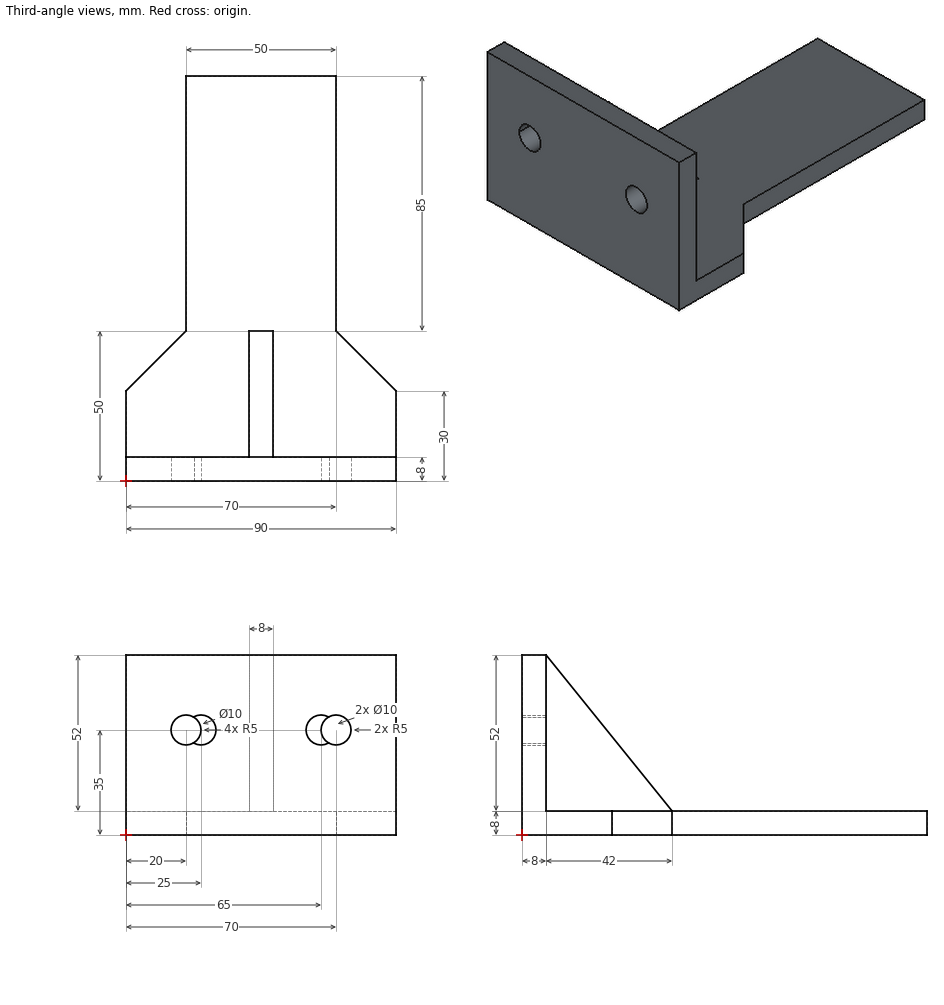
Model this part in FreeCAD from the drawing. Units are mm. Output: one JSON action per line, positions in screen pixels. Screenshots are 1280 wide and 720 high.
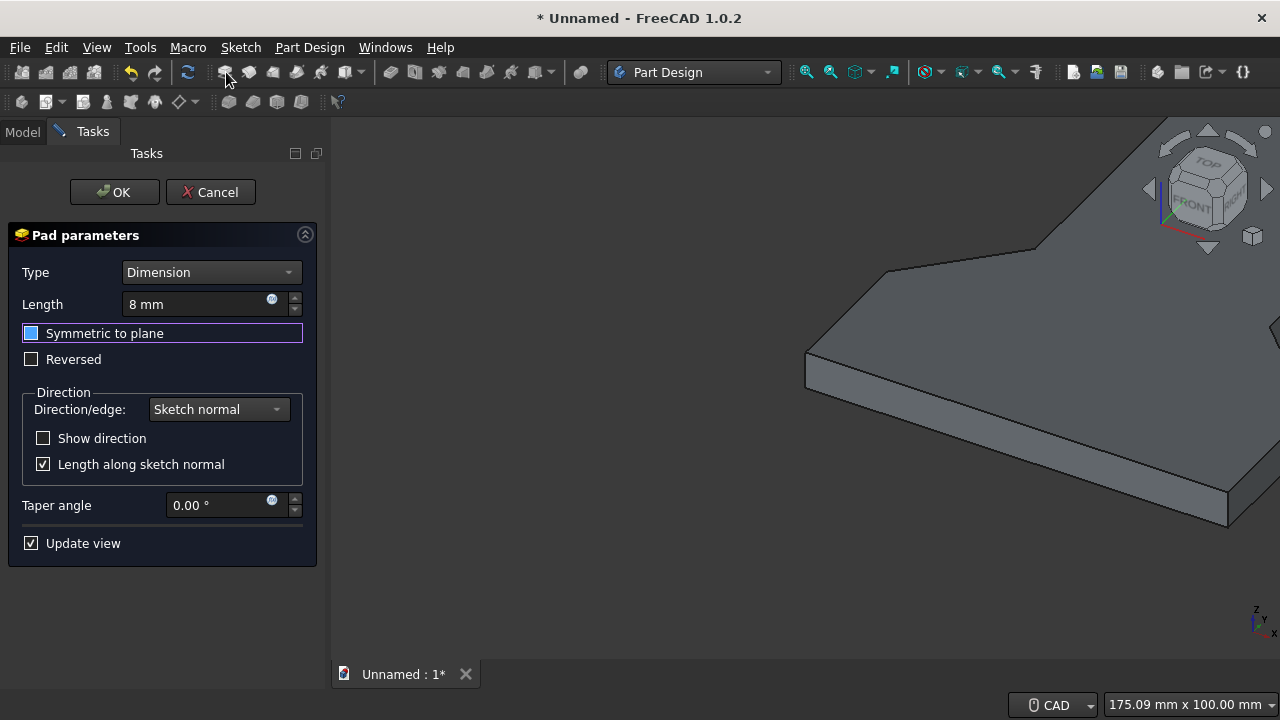
{"action": "left_click", "coordinate": [115, 192]}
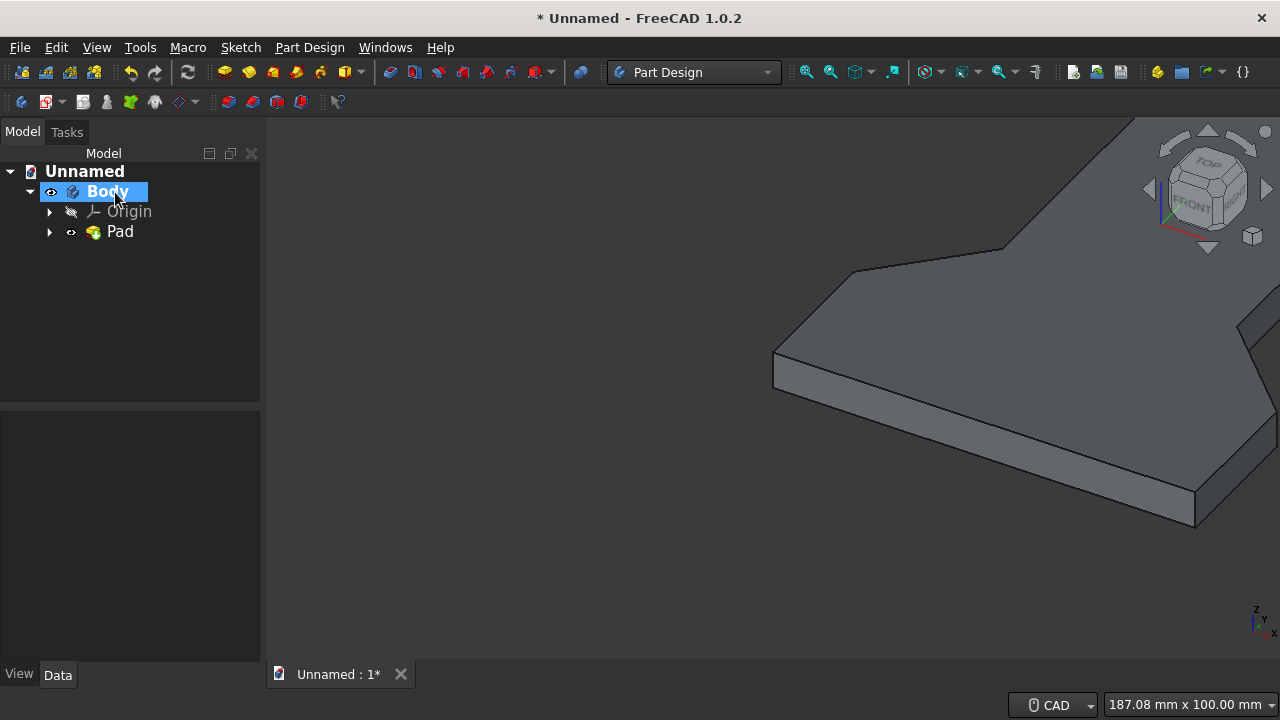
{"action": "left_click", "coordinate": [808, 72]}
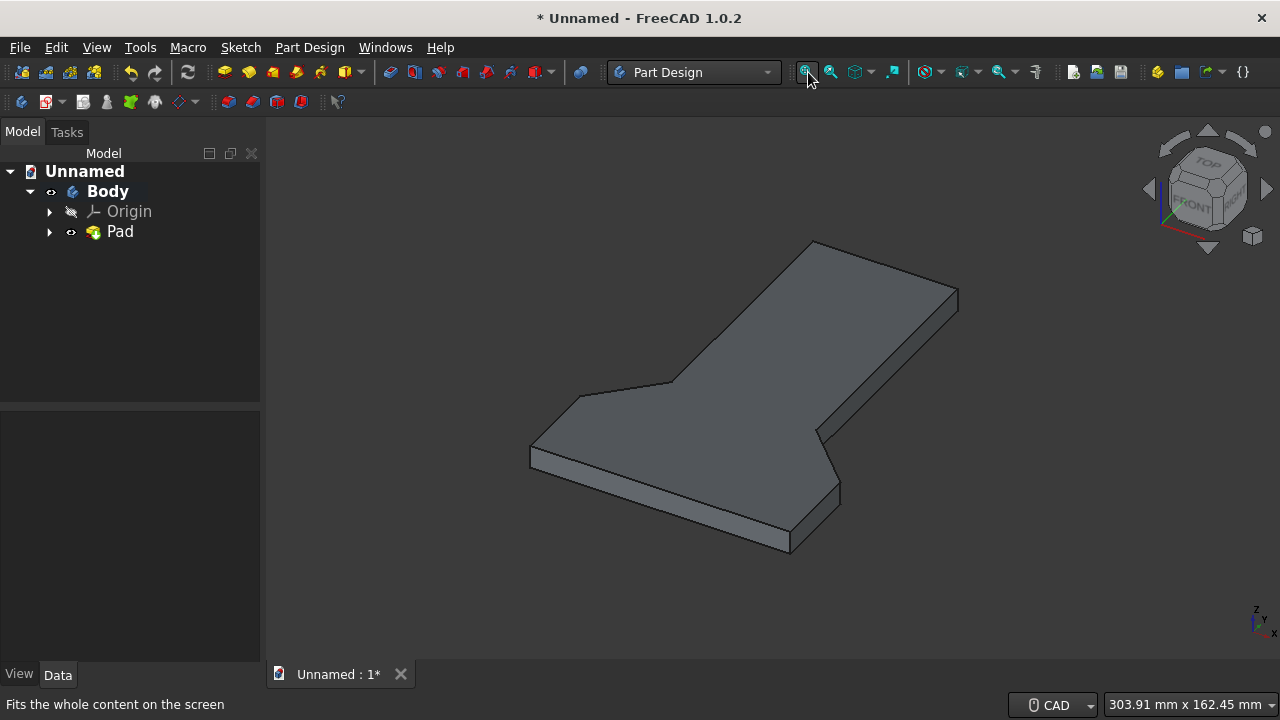
{"action": "left_click", "coordinate": [709, 440]}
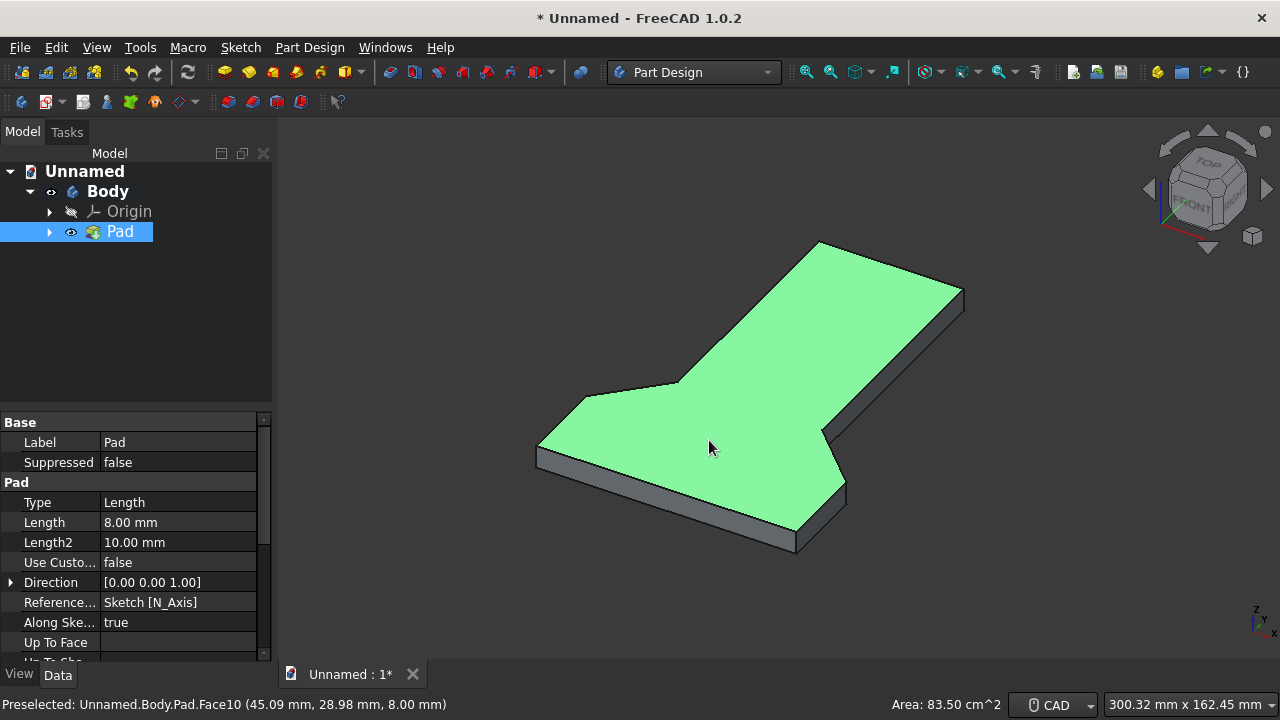
{"action": "left_click", "coordinate": [46, 102]}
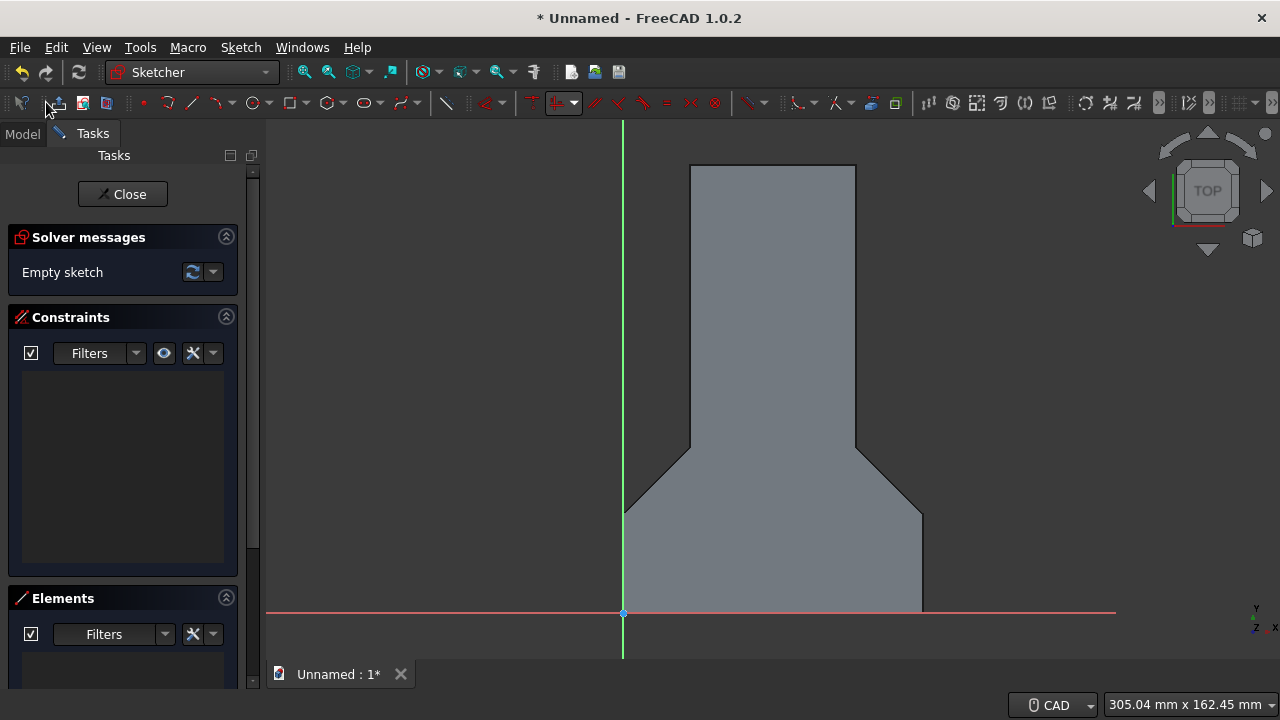
{"action": "scroll", "coordinate": [856, 631], "scroll_direction": "up", "scroll_amount": 3}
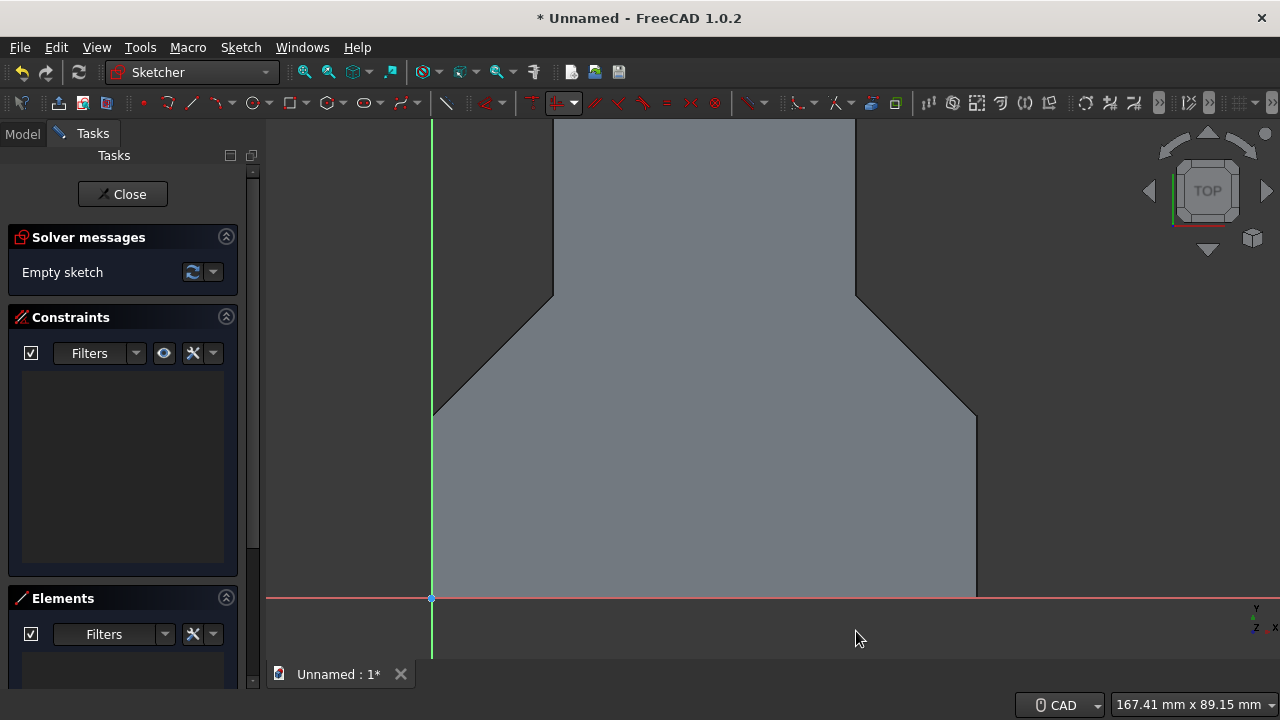
{"action": "left_click", "coordinate": [290, 104]}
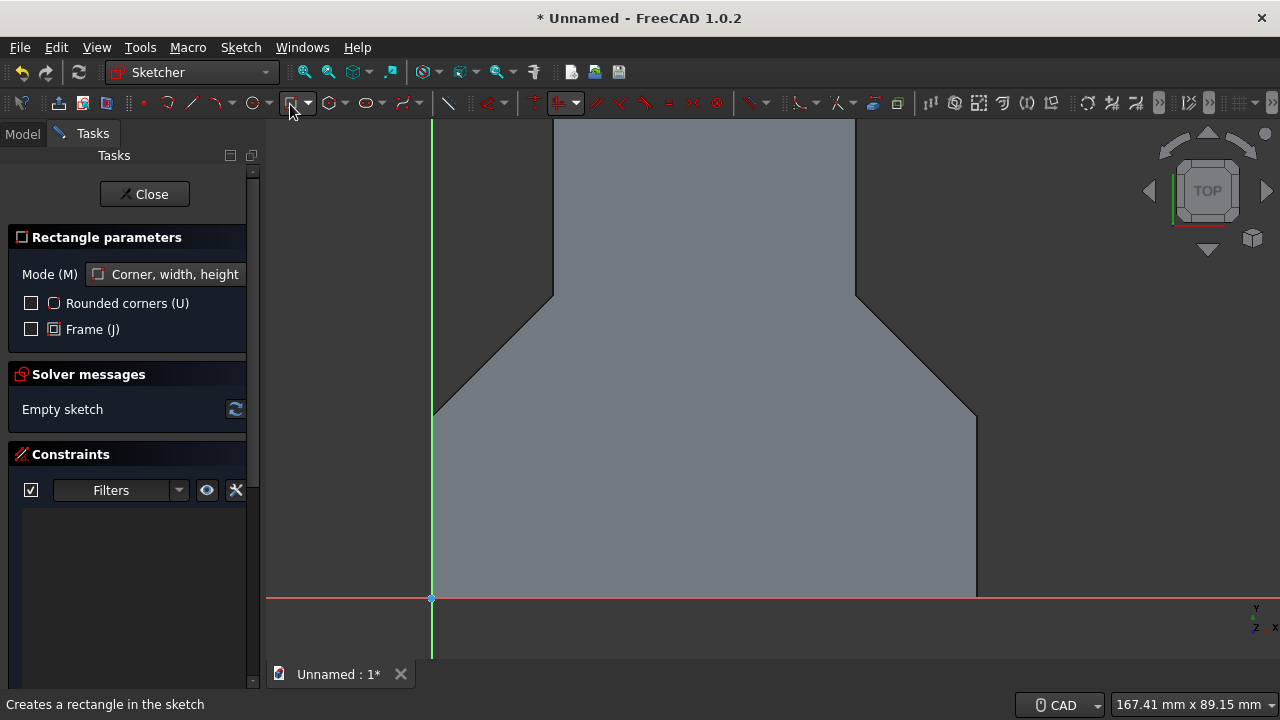
{"action": "left_click", "coordinate": [432, 598]}
{"action": "mouse_move", "coordinate": [977, 550]}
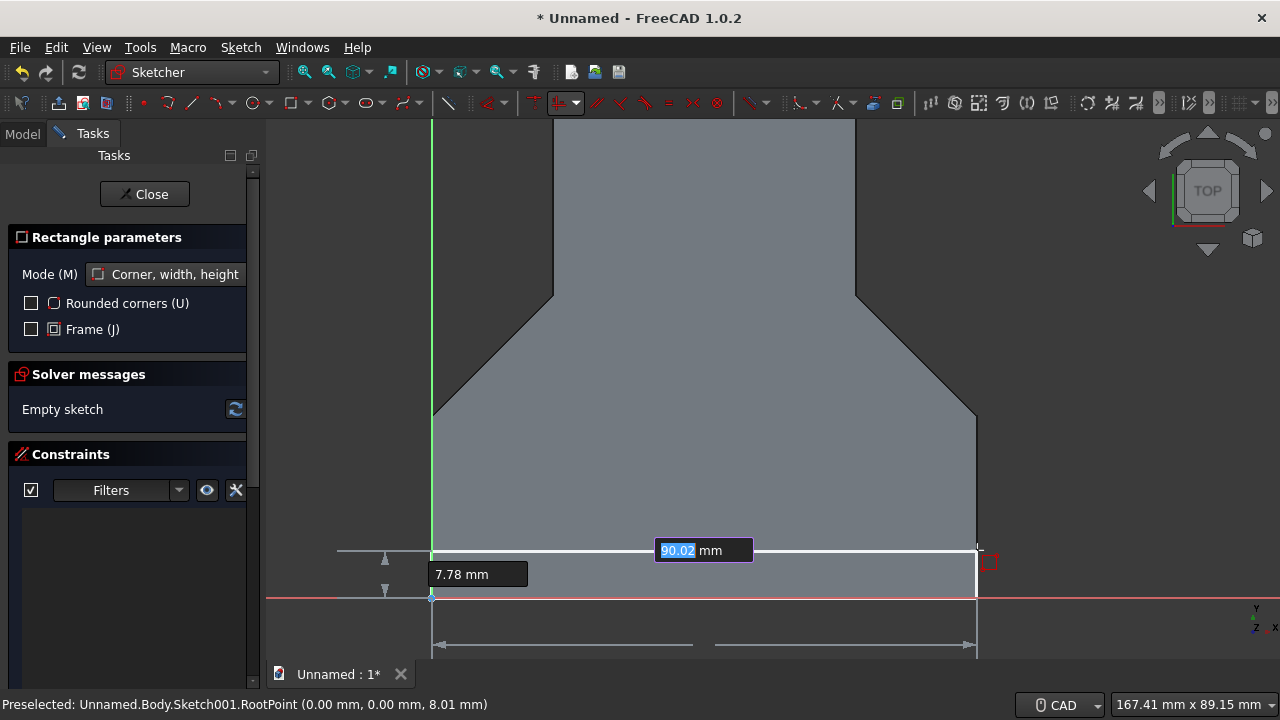
{"action": "type", "text": "90"}
{"action": "key", "text": "Tab"}
{"action": "type", "text": "8"}
{"action": "key", "text": "Return"}
{"action": "key", "text": "Escape"}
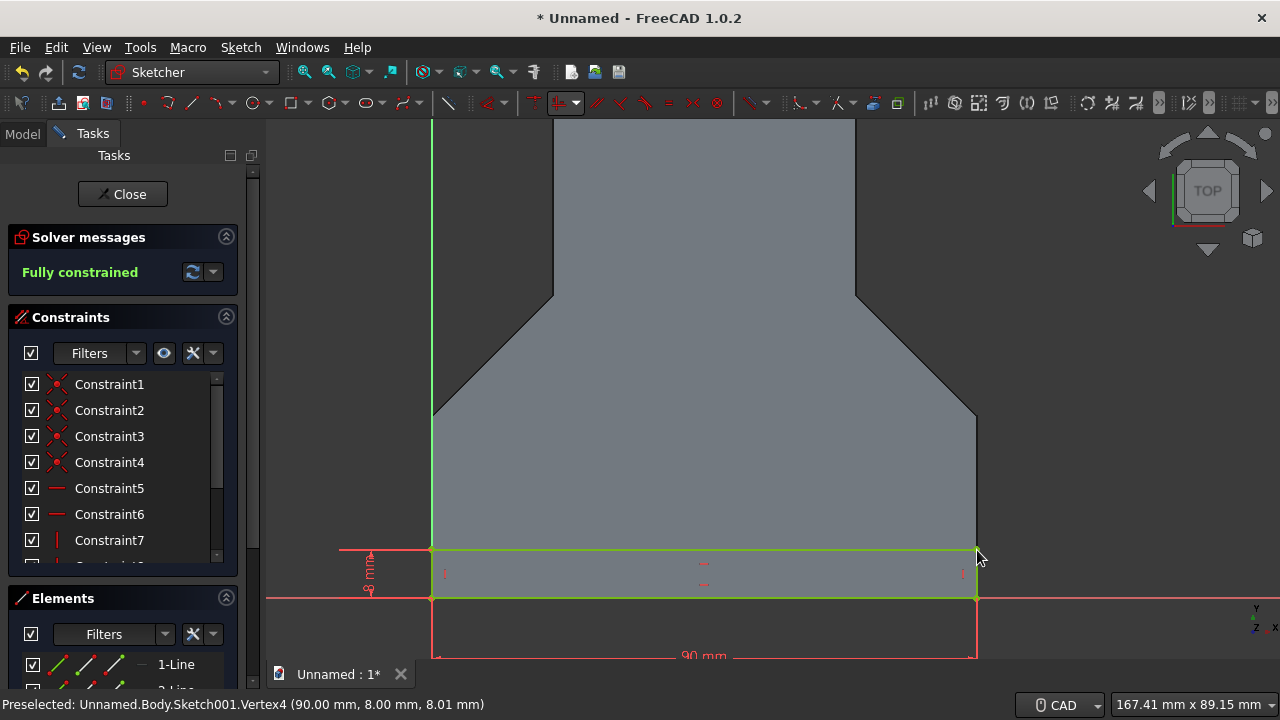
{"action": "left_click", "coordinate": [123, 194]}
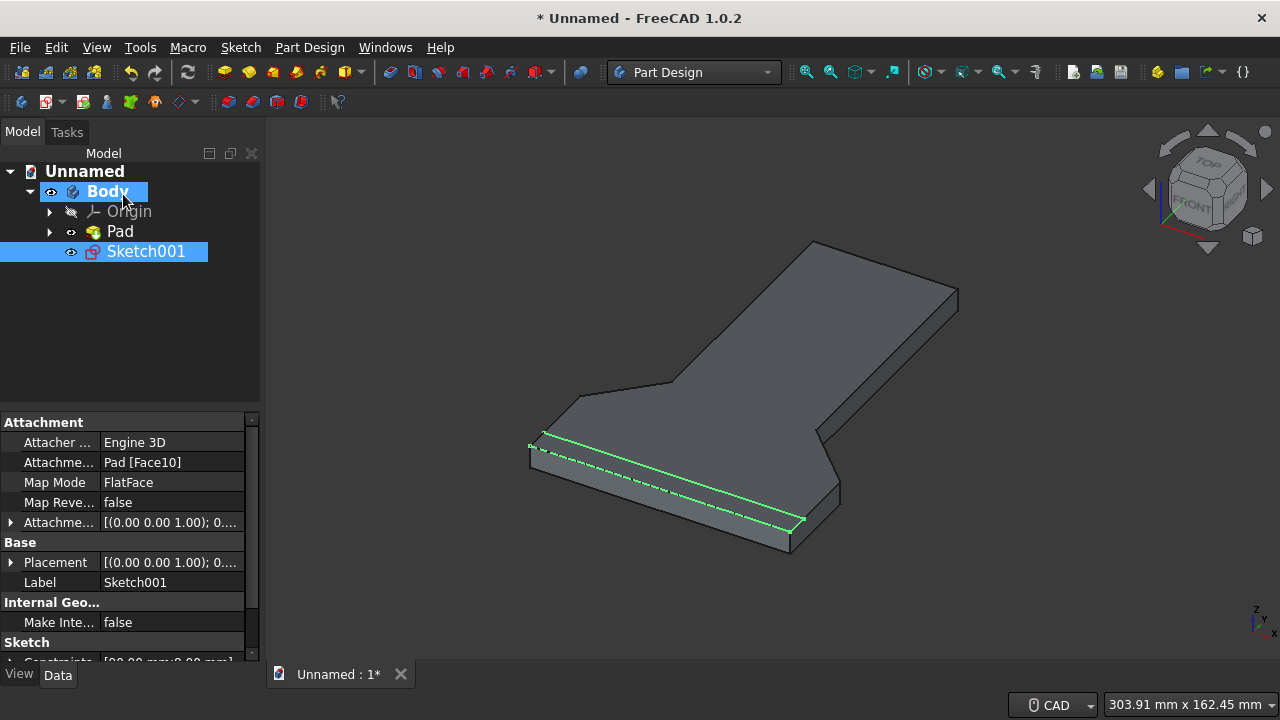
{"action": "left_click", "coordinate": [226, 72]}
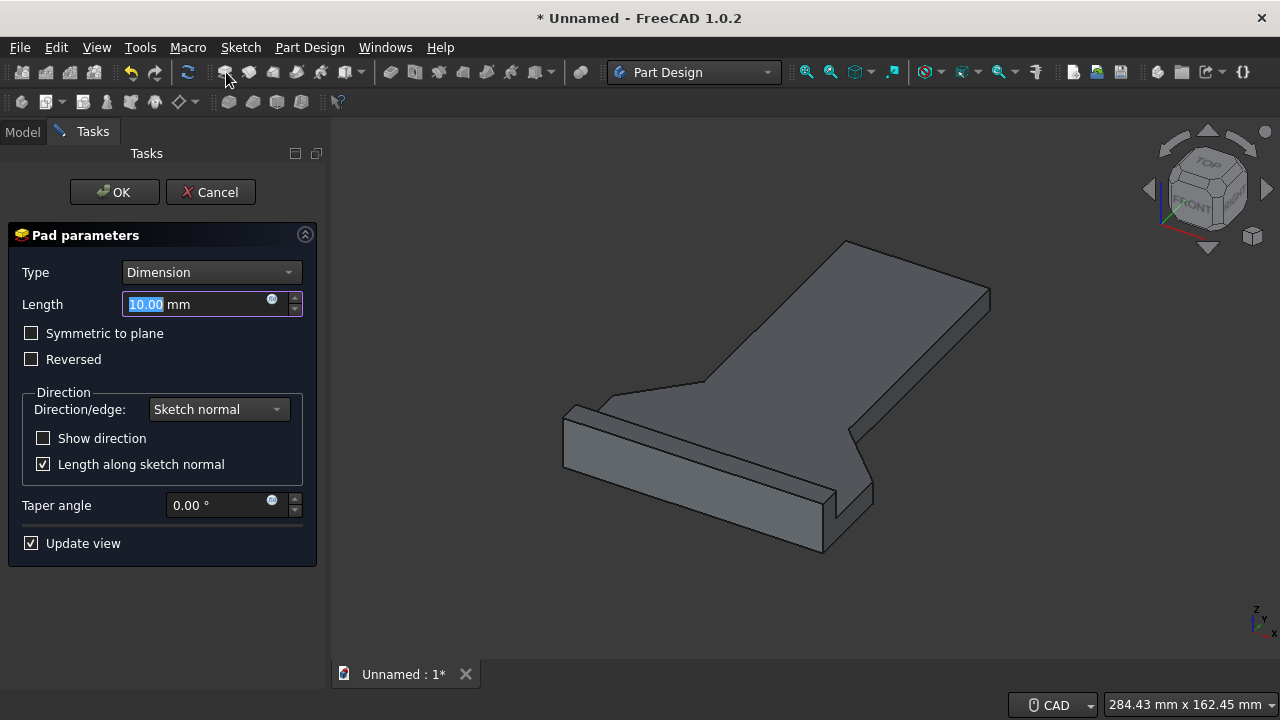
{"action": "type", "text": "52"}
{"action": "key", "text": "Tab"}